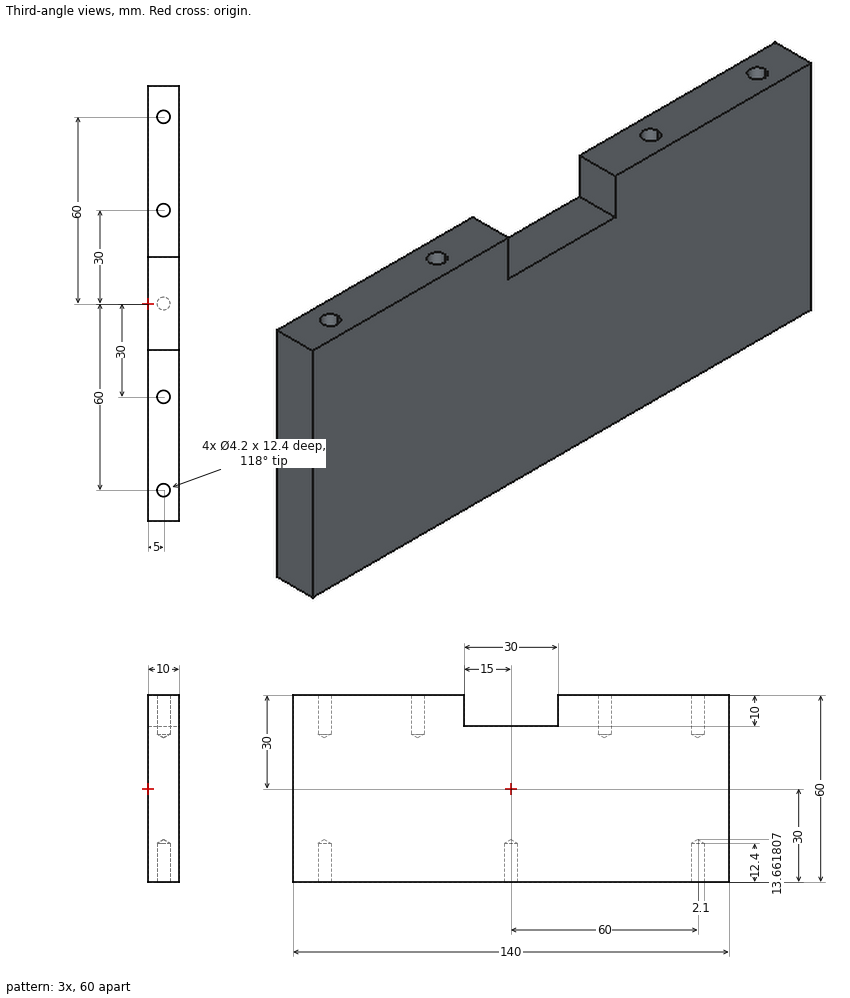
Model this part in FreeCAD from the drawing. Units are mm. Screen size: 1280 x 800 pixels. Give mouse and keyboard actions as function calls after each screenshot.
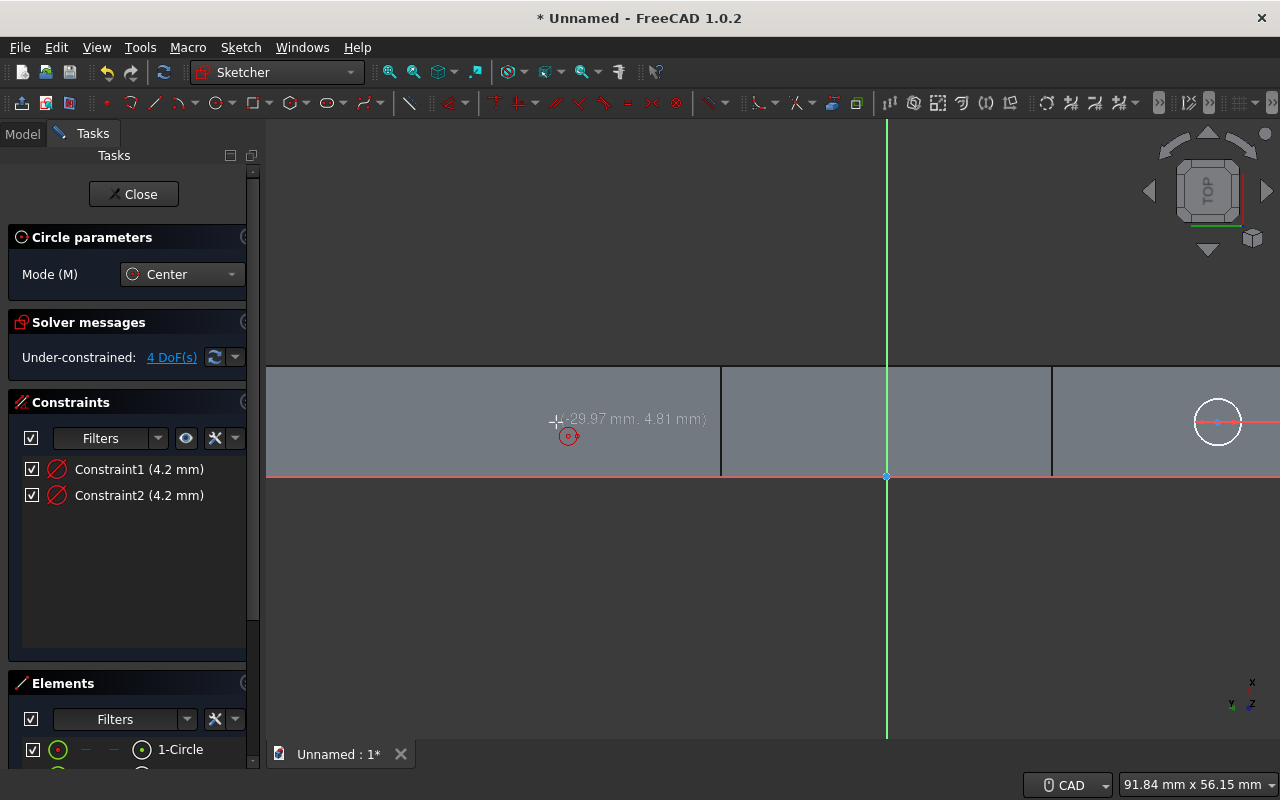
click(555, 422)
move(572, 405)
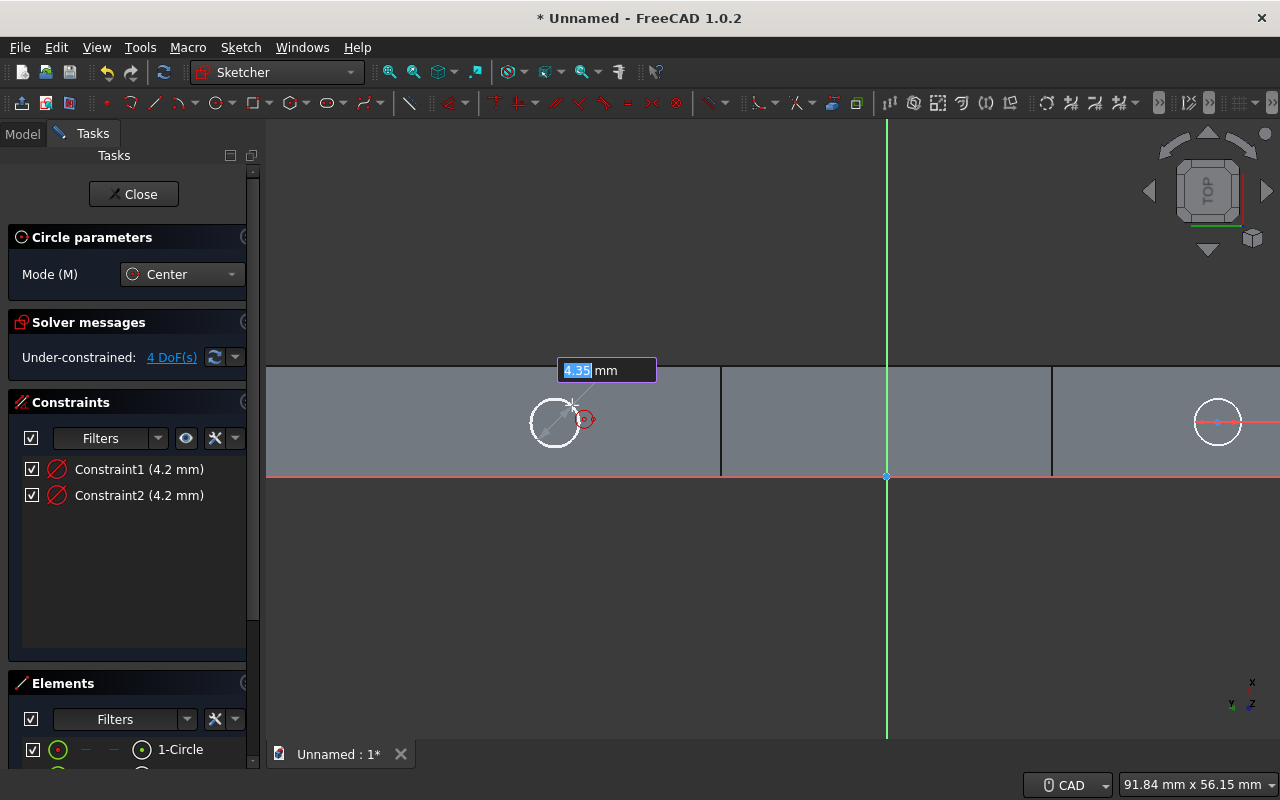
text(4.2)
key(Return)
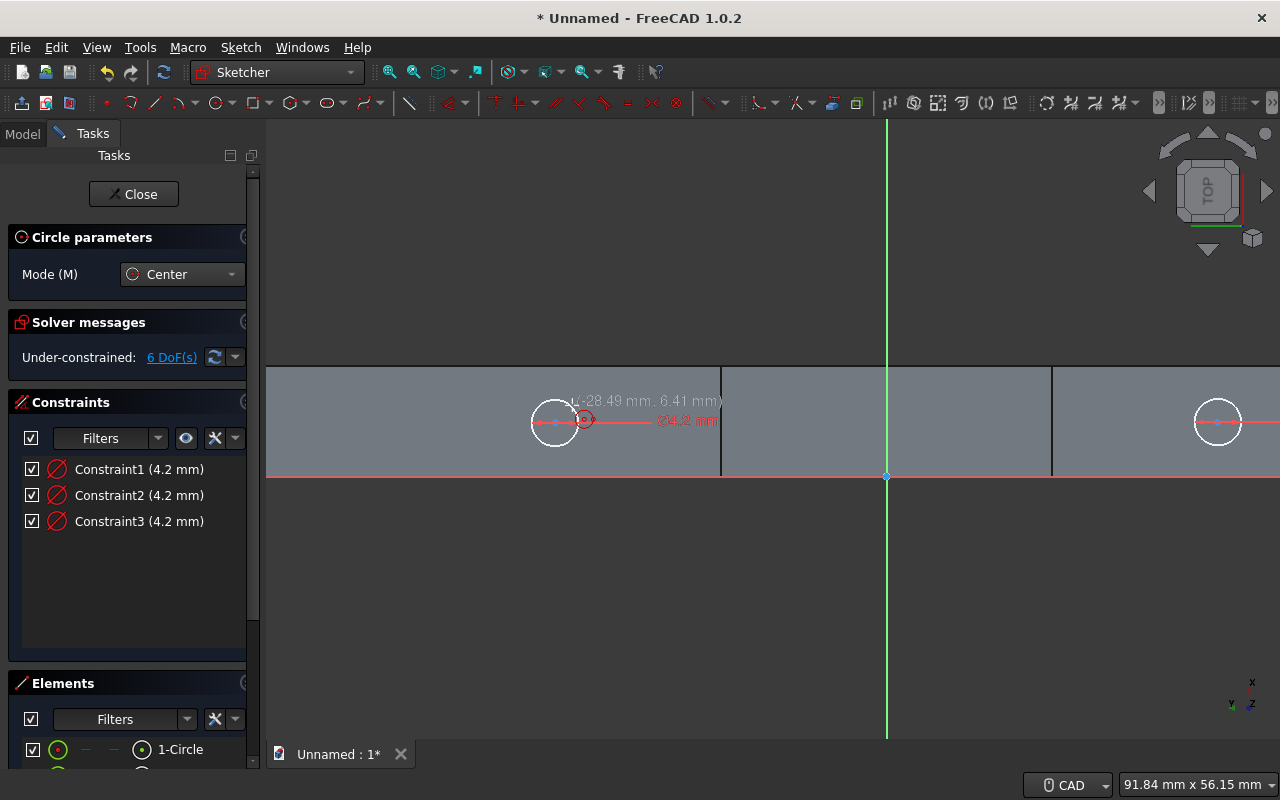
scroll(556, 422, down, 4)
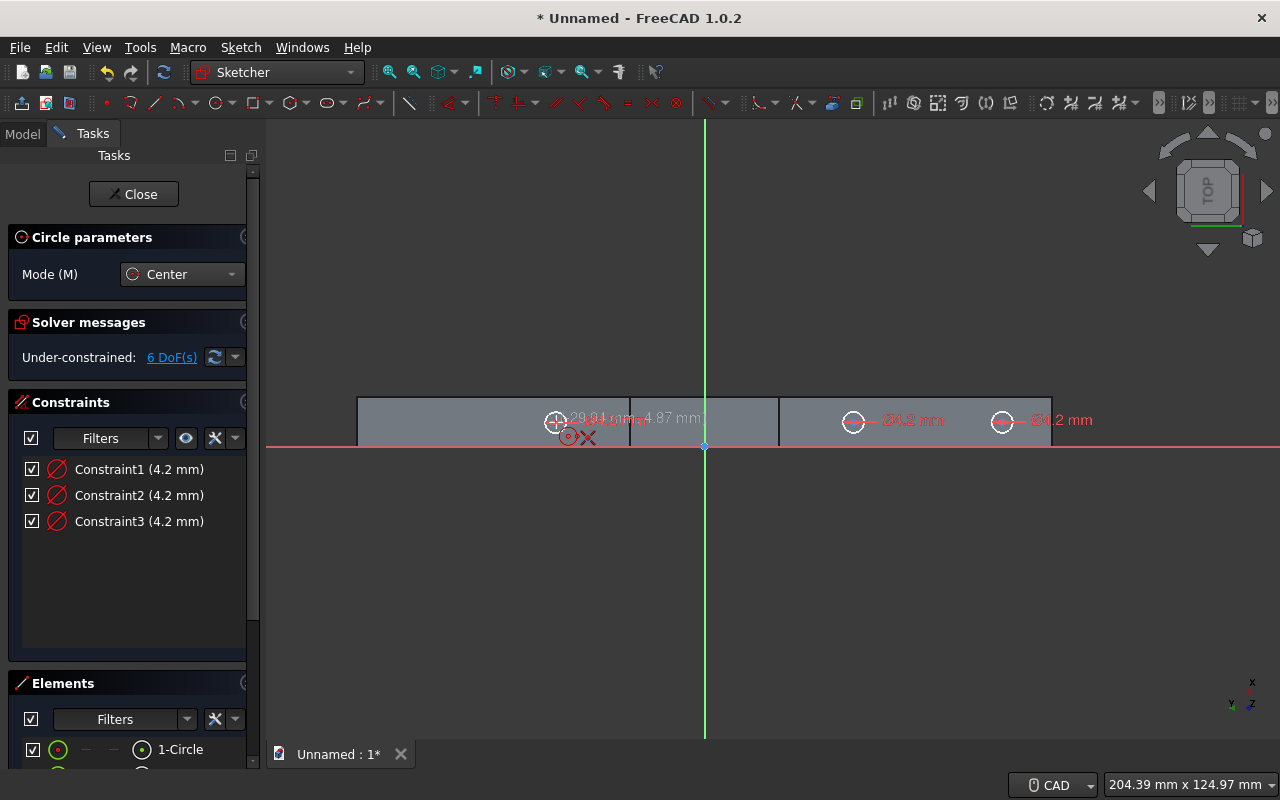
scroll(407, 422, up, 4)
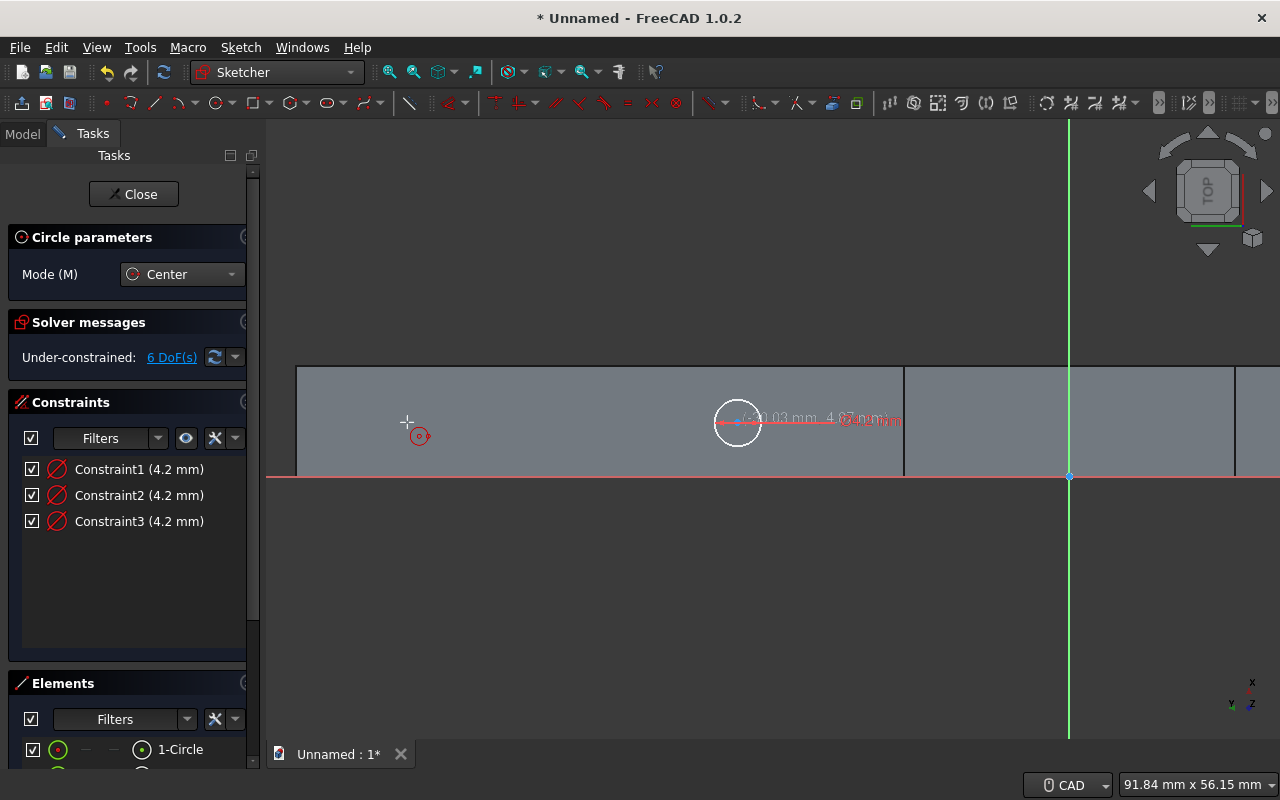
click(407, 422)
move(423, 405)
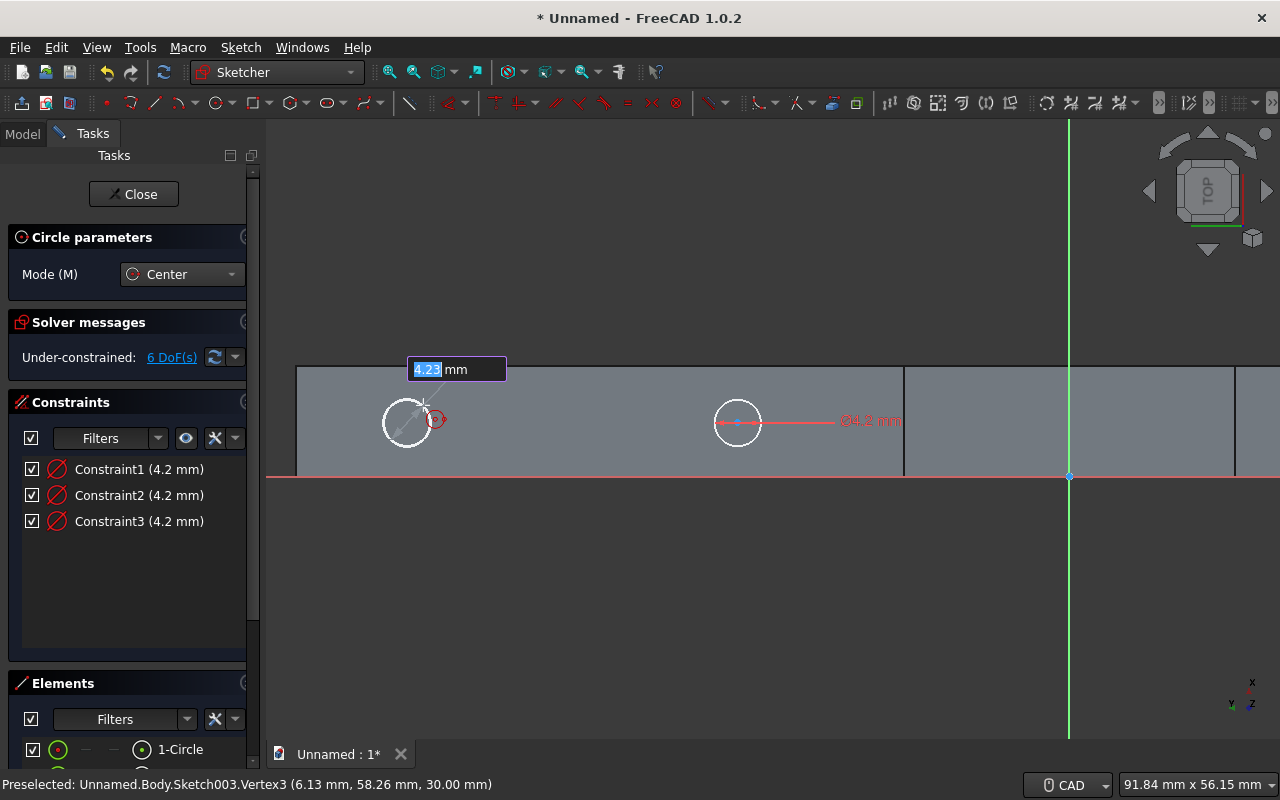
text(4.2)
key(Return)
key(Escape)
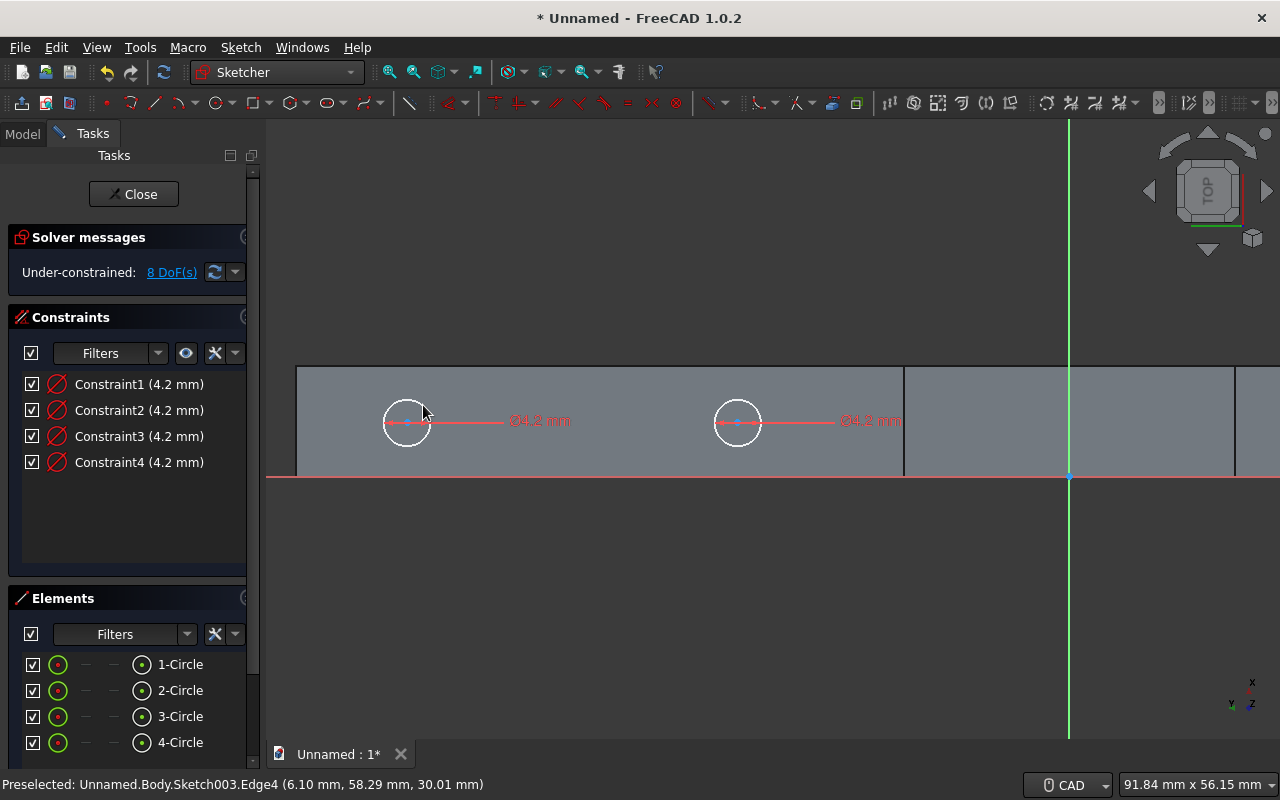
scroll(407, 422, down, 4)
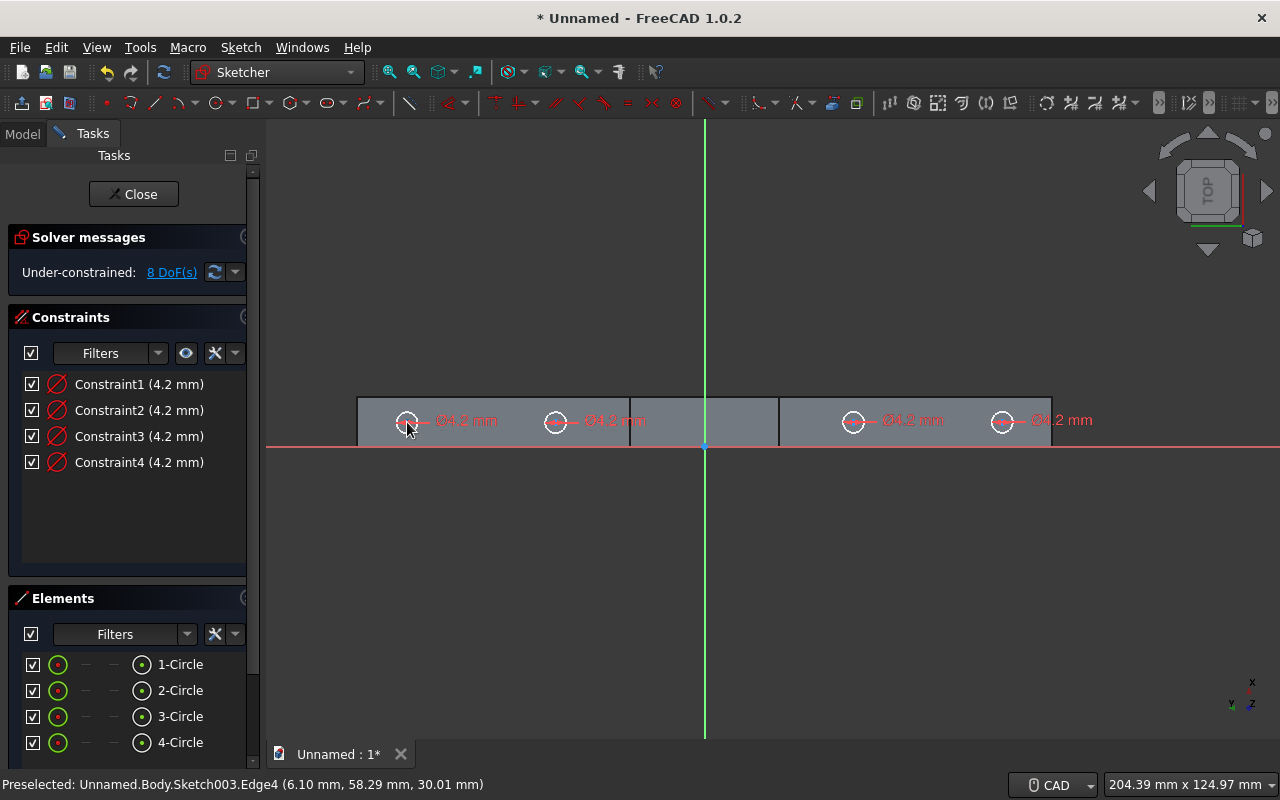
click(1002, 422)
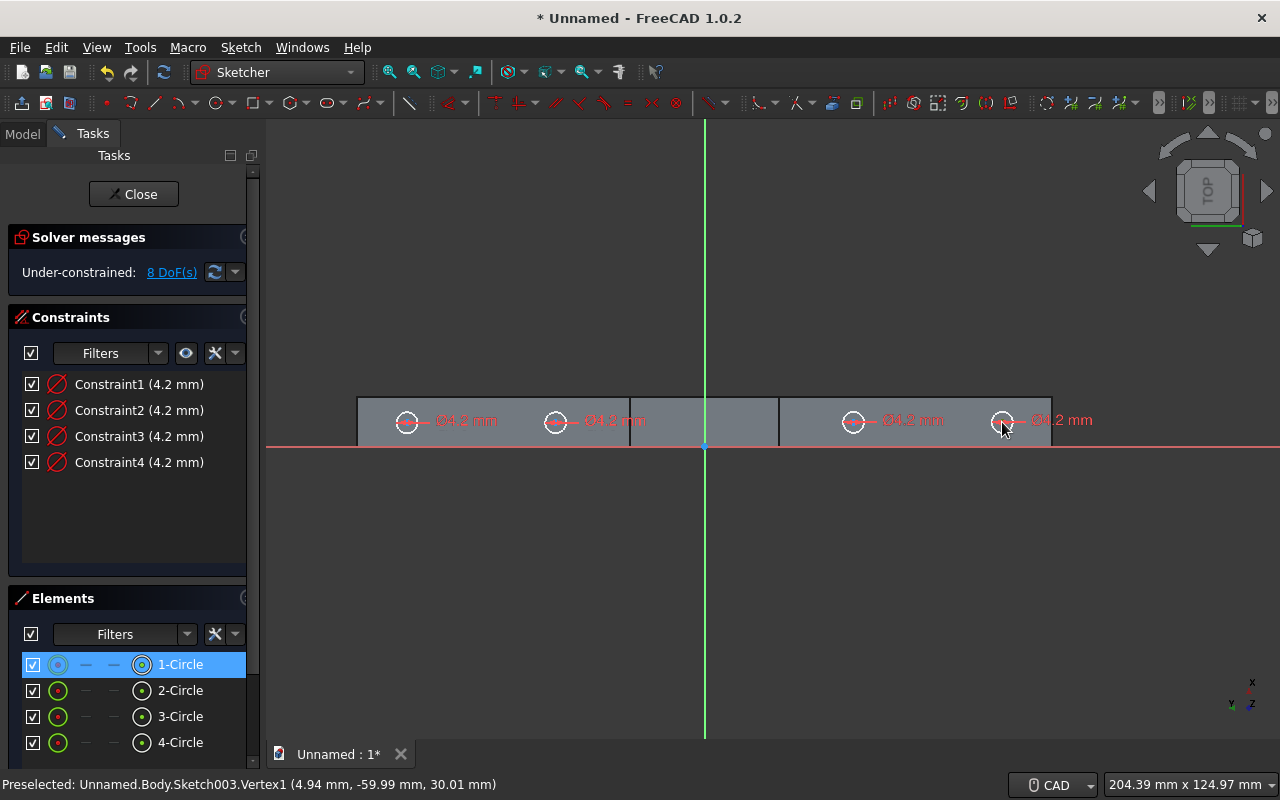
click(854, 422)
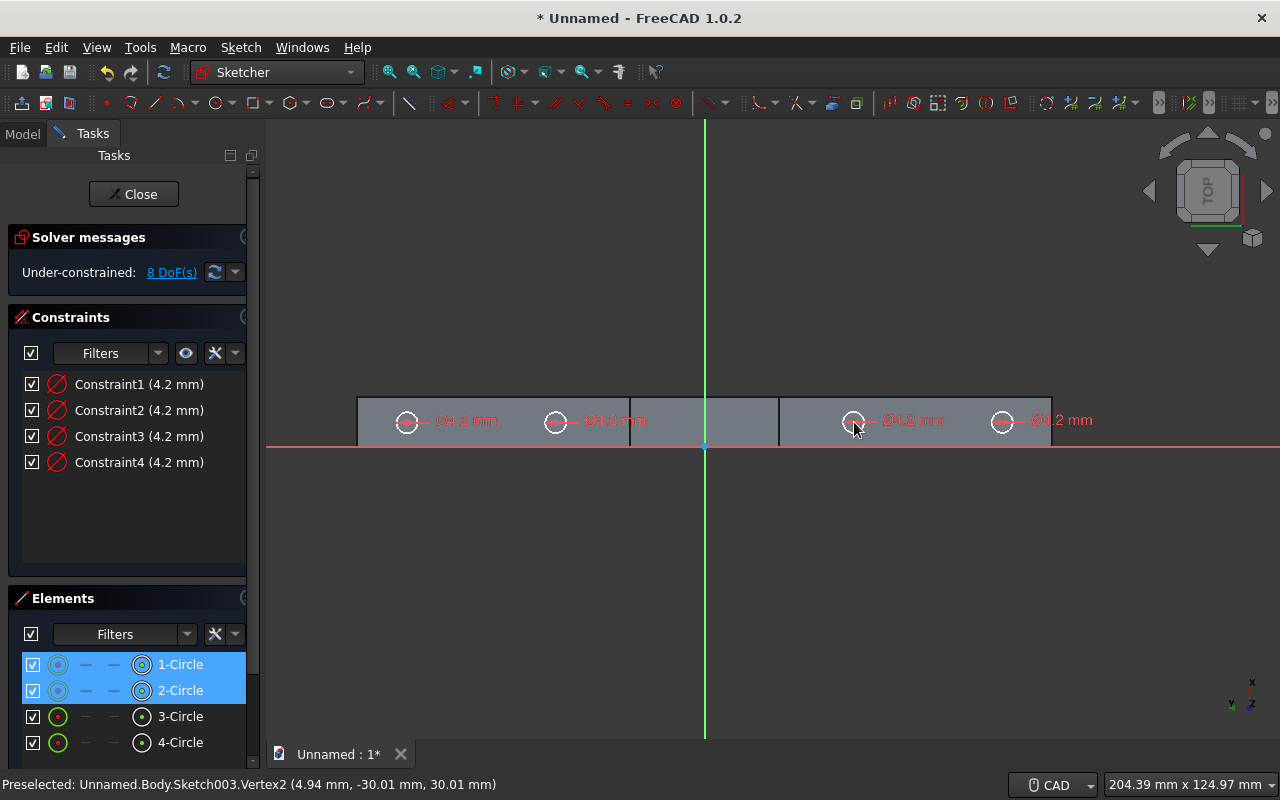
key(h)